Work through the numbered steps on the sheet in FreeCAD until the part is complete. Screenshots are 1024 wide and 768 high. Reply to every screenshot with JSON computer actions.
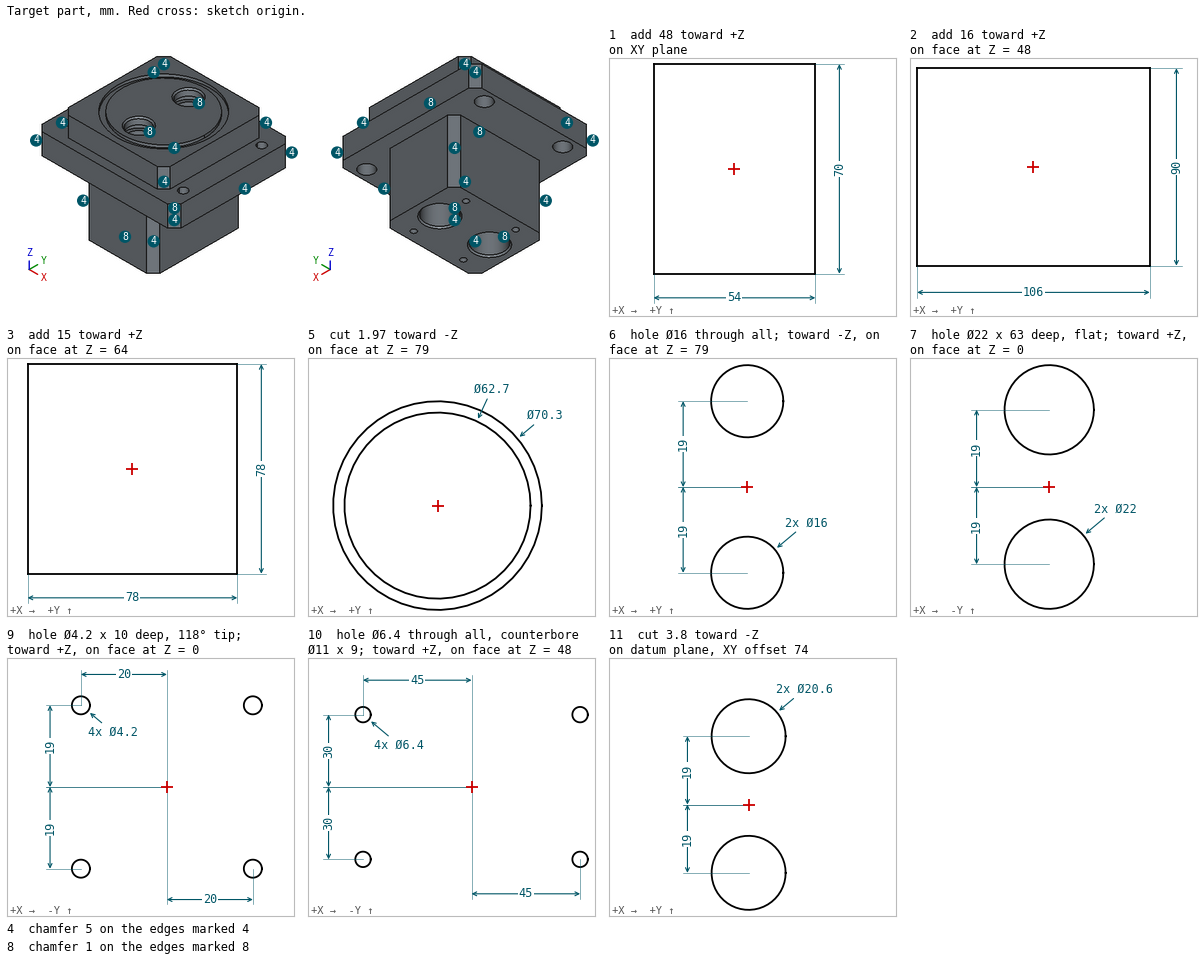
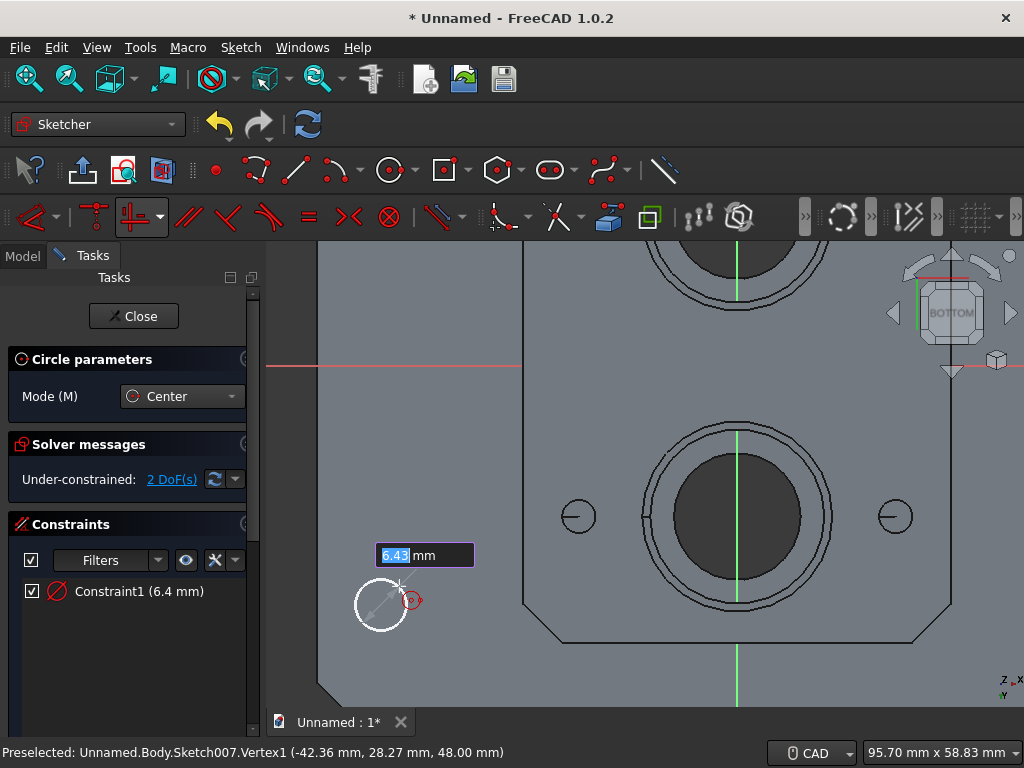
{"action": "type", "text": "6.4"}
{"action": "key", "text": "Return"}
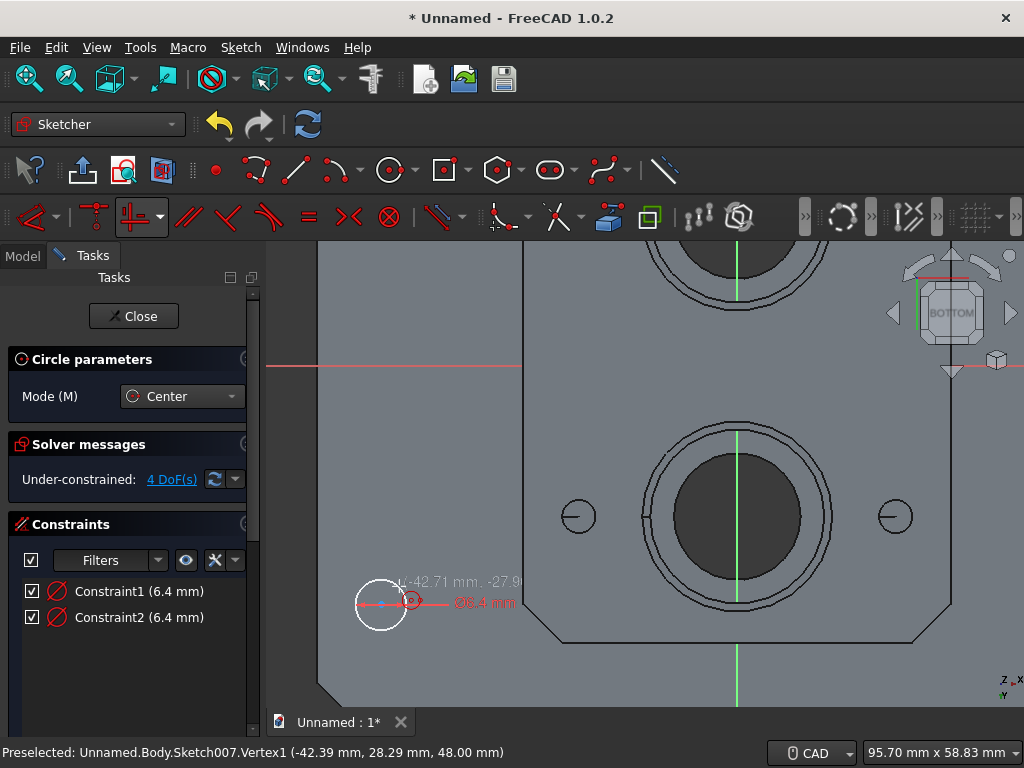
{"action": "scroll", "coordinate": [381, 605], "scroll_direction": "down", "scroll_amount": 3}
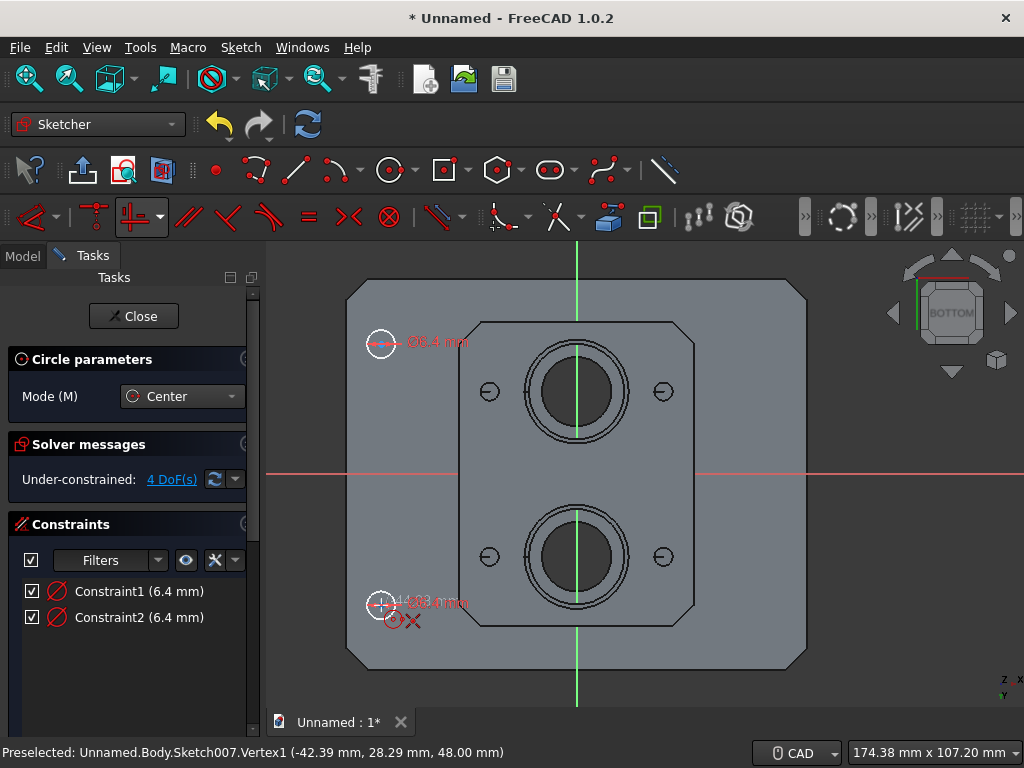
{"action": "scroll", "coordinate": [772, 605], "scroll_direction": "up", "scroll_amount": 3}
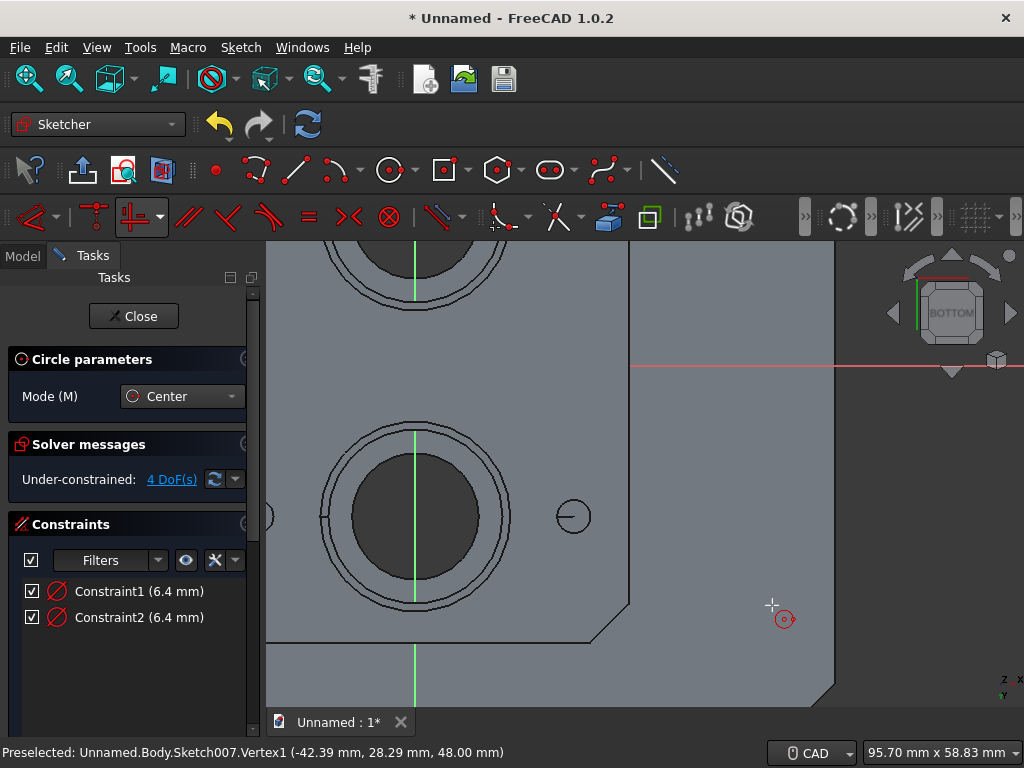
{"action": "left_click", "coordinate": [772, 604]}
{"action": "mouse_move", "coordinate": [790, 586]}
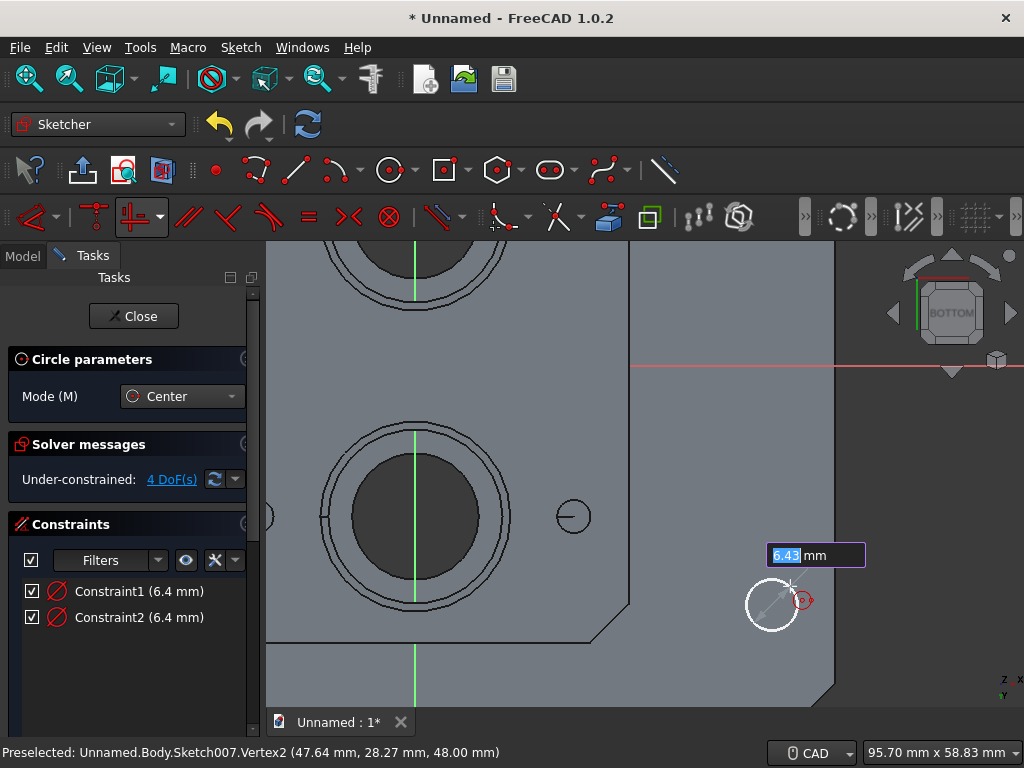
{"action": "type", "text": "6.4"}
{"action": "key", "text": "Return"}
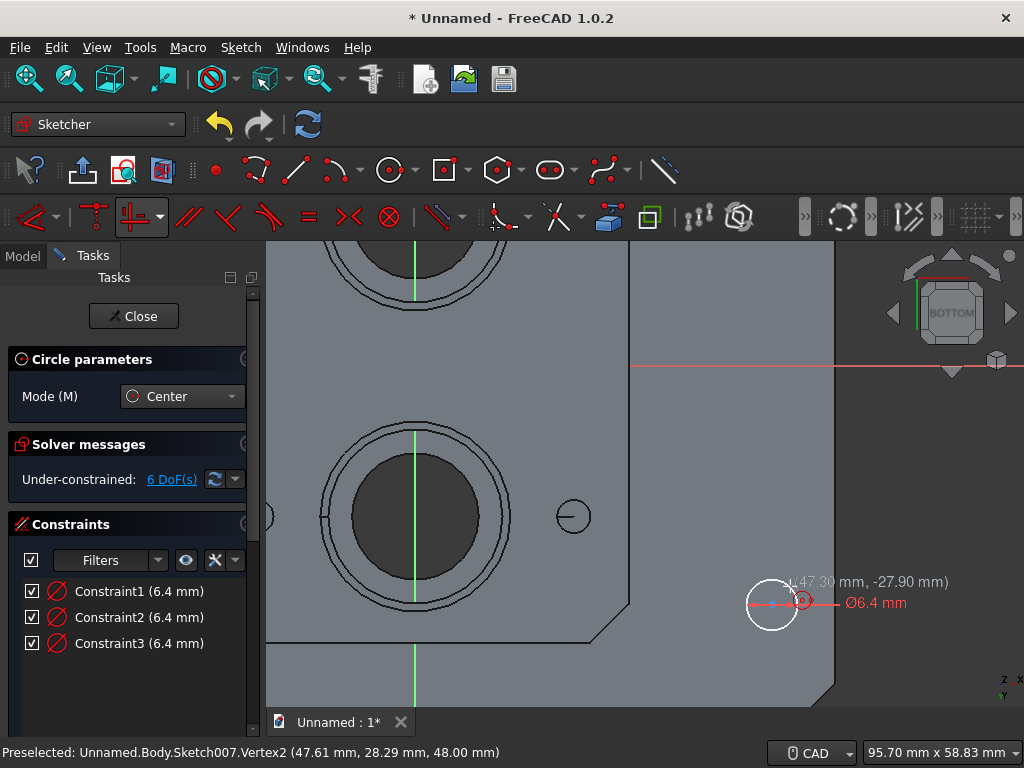
{"action": "scroll", "coordinate": [772, 605], "scroll_direction": "down", "scroll_amount": 3}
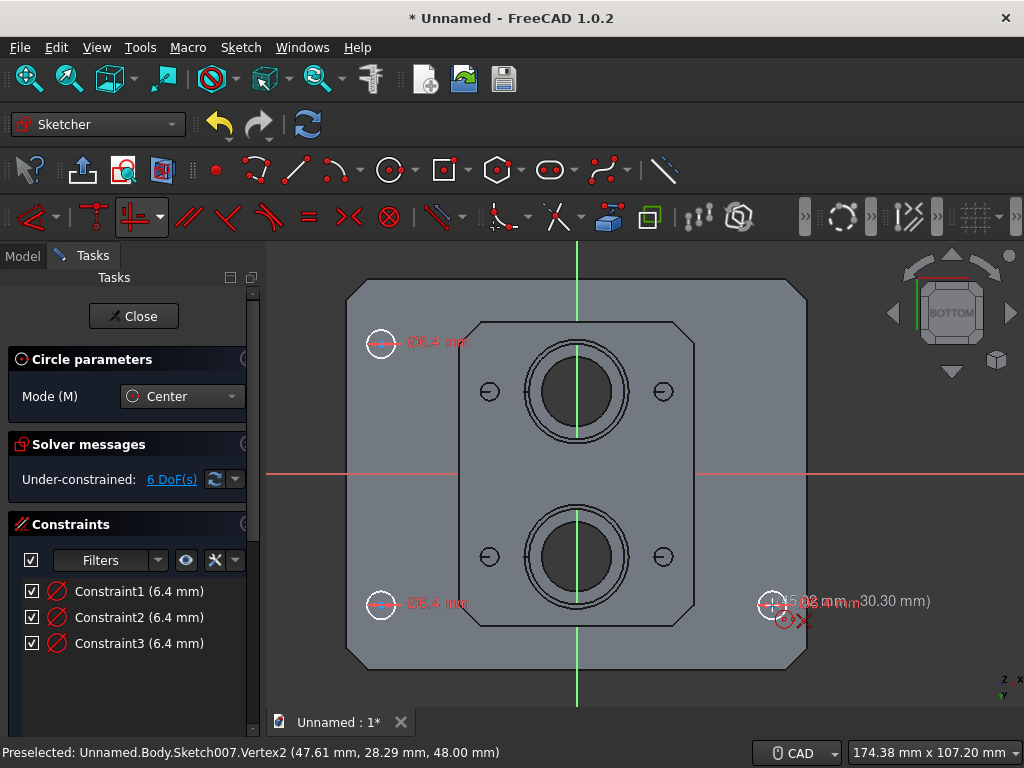
{"action": "scroll", "coordinate": [772, 344], "scroll_direction": "up", "scroll_amount": 3}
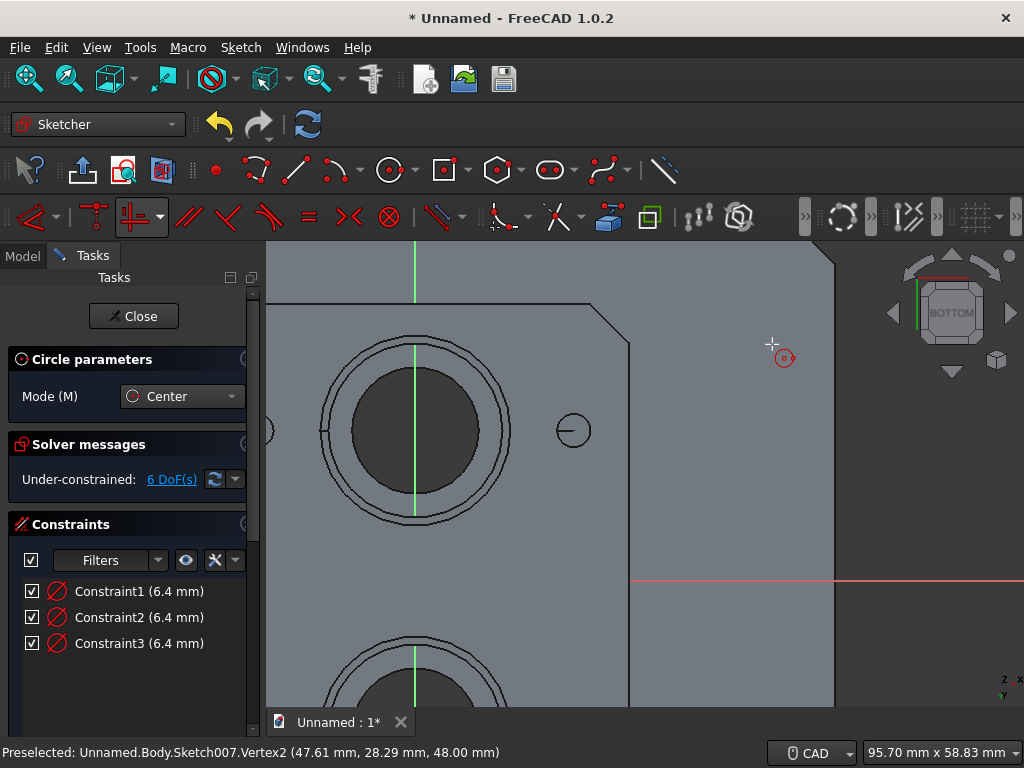
{"action": "left_click", "coordinate": [772, 343]}
{"action": "mouse_move", "coordinate": [790, 326]}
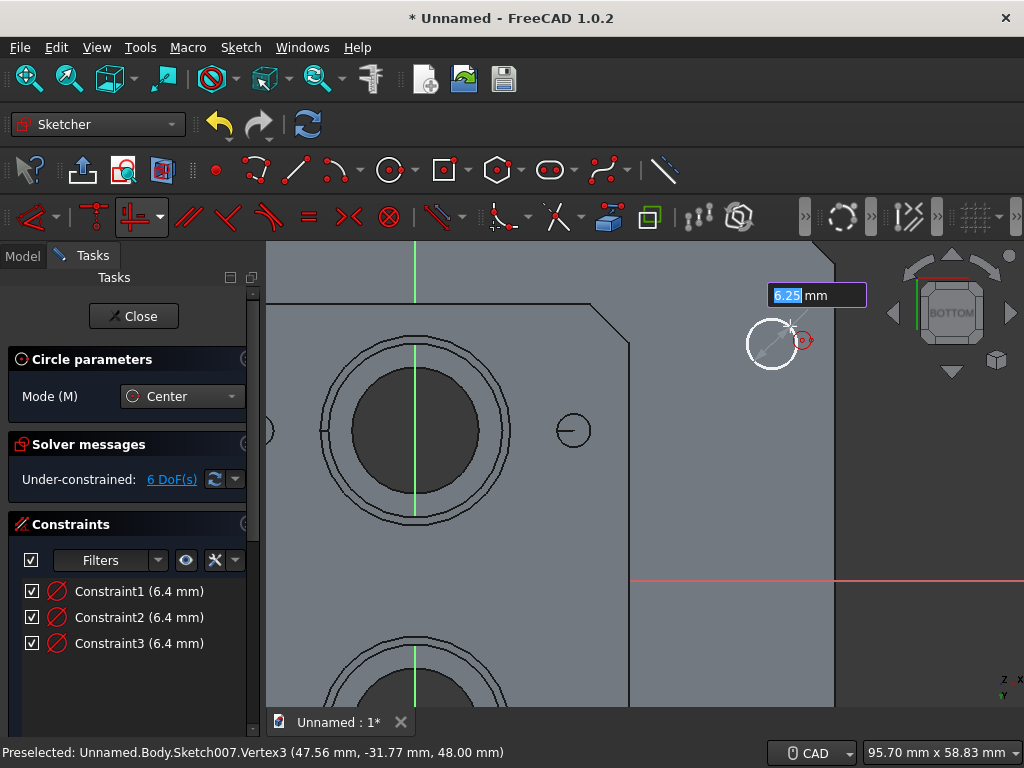
{"action": "type", "text": "6.4"}
{"action": "key", "text": "Return"}
{"action": "key", "text": "Escape"}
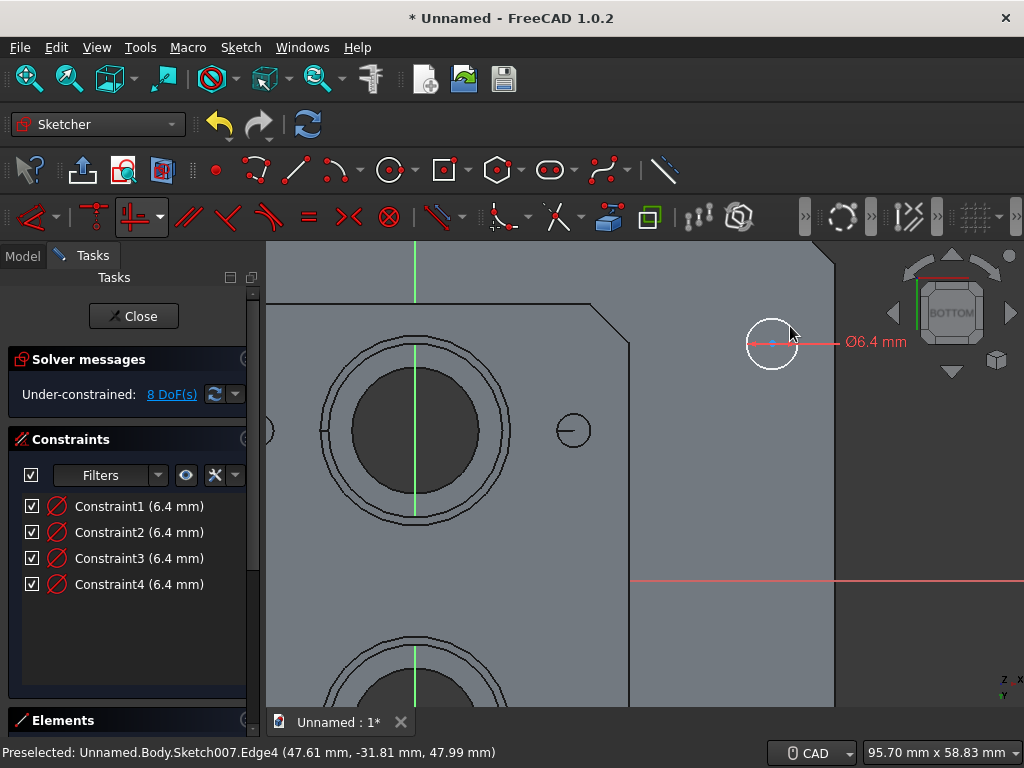
{"action": "scroll", "coordinate": [772, 344], "scroll_direction": "down", "scroll_amount": 3}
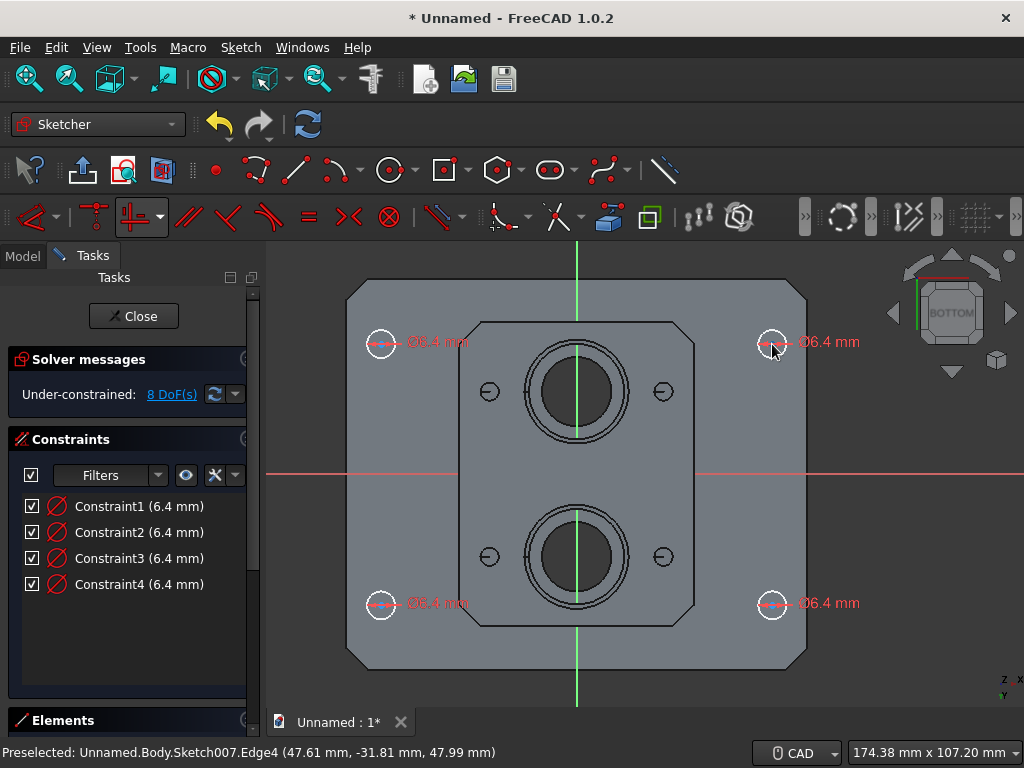
{"action": "left_click", "coordinate": [381, 344]}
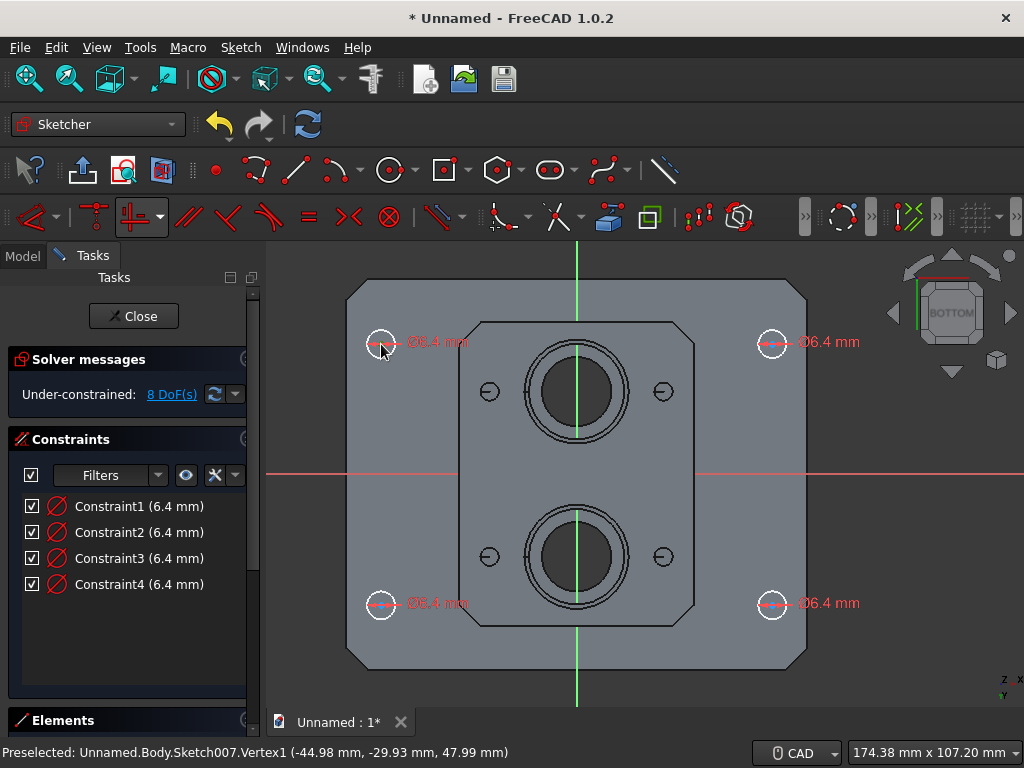
{"action": "left_click", "coordinate": [381, 605]}